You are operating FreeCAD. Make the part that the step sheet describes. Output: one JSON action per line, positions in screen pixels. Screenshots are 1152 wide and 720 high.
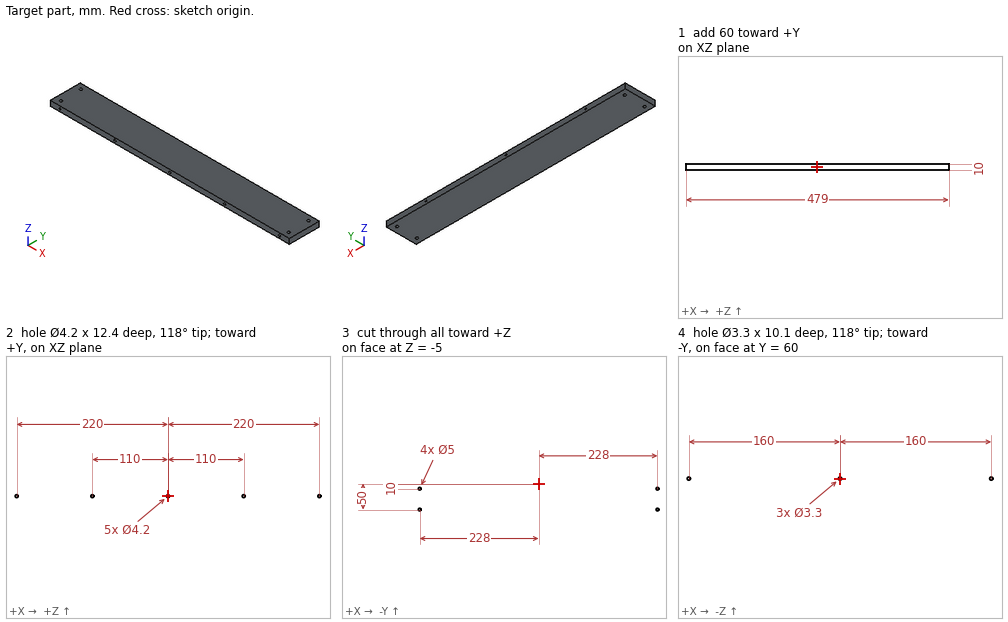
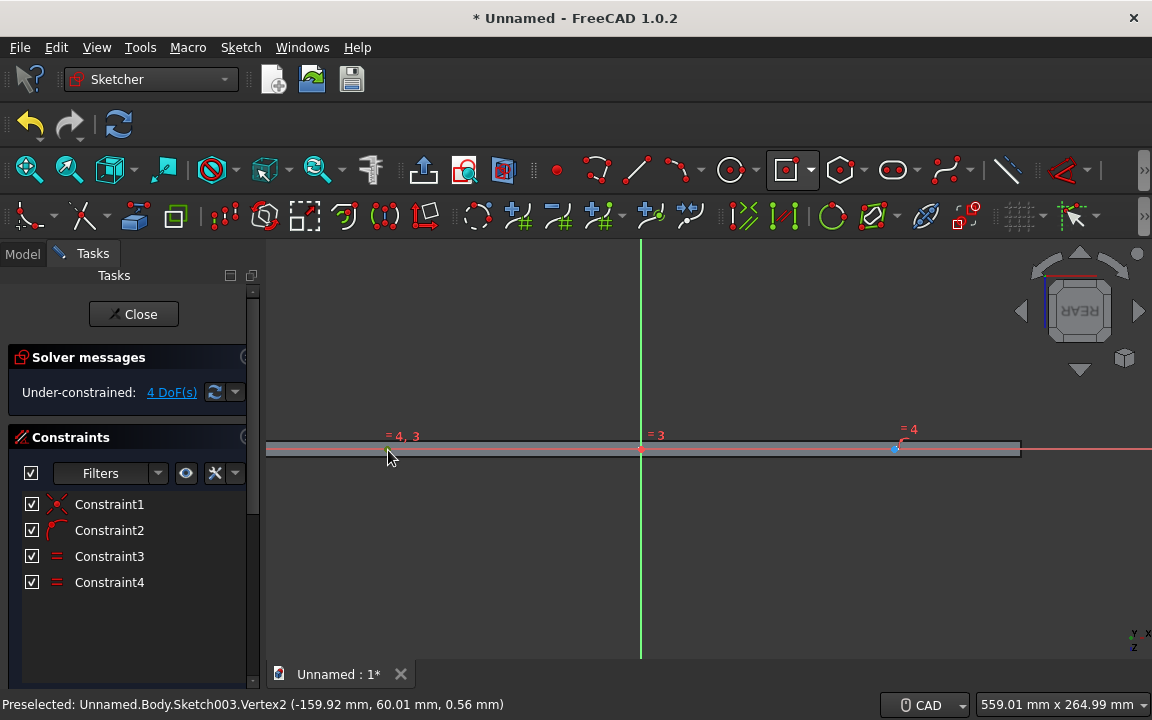
{"action": "left_click", "coordinate": [344, 449]}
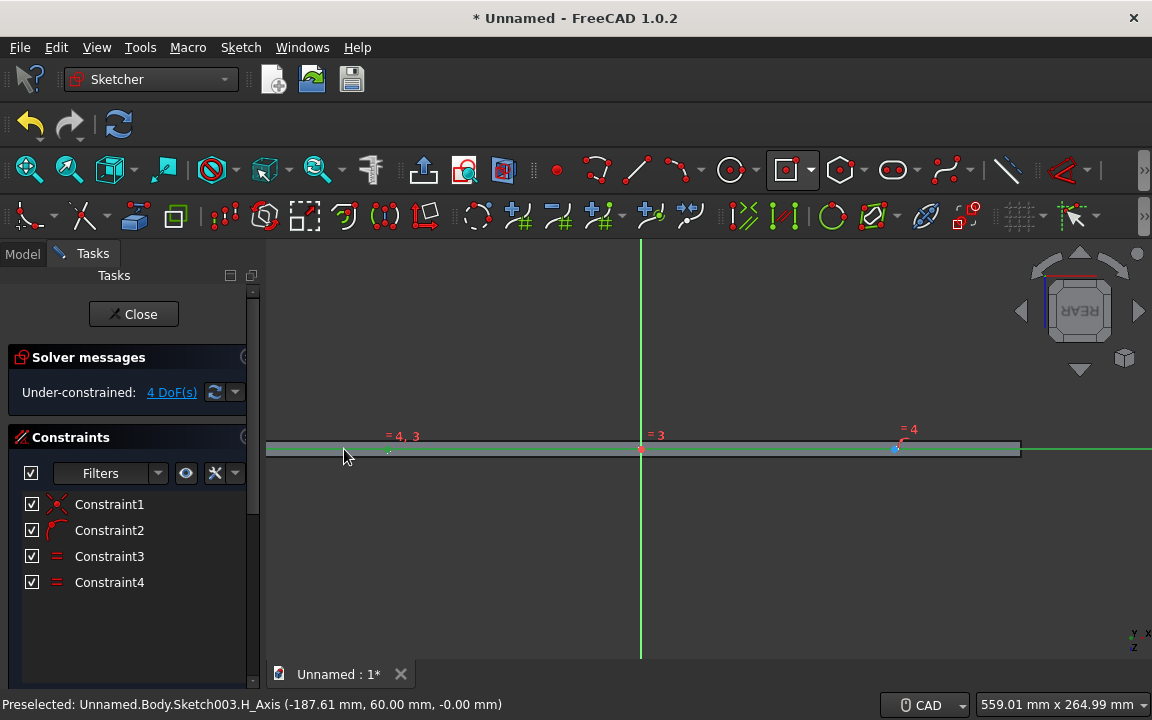
{"action": "key", "text": "c"}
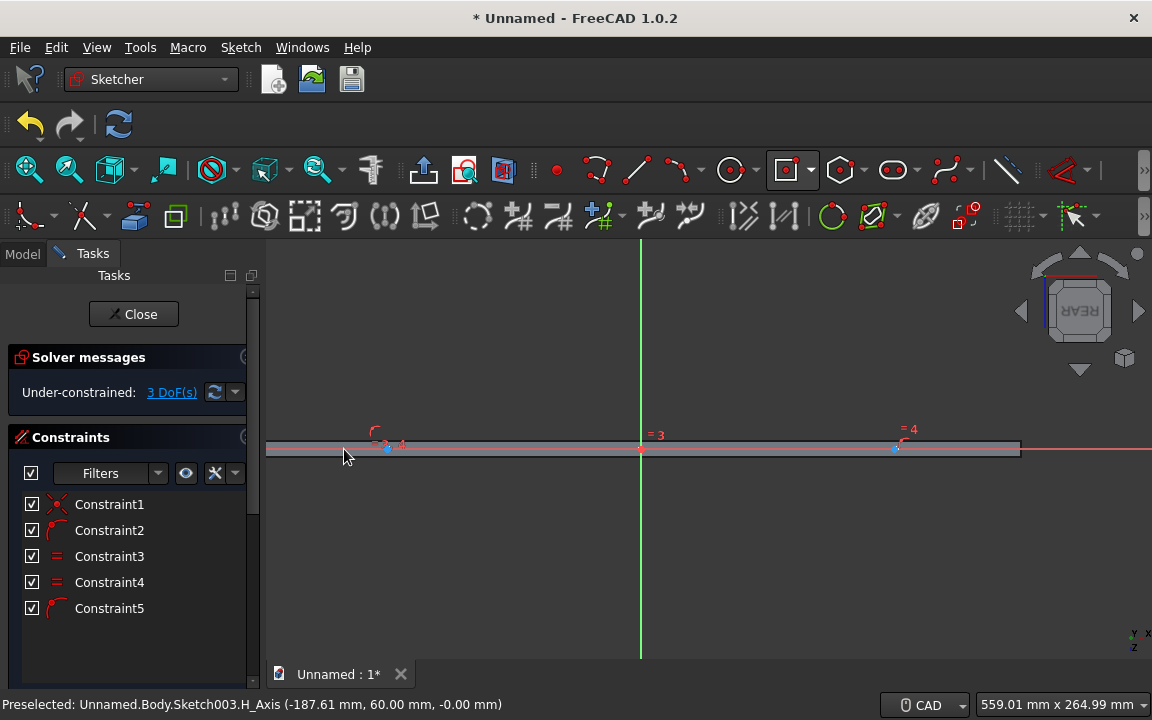
{"action": "key", "text": "d"}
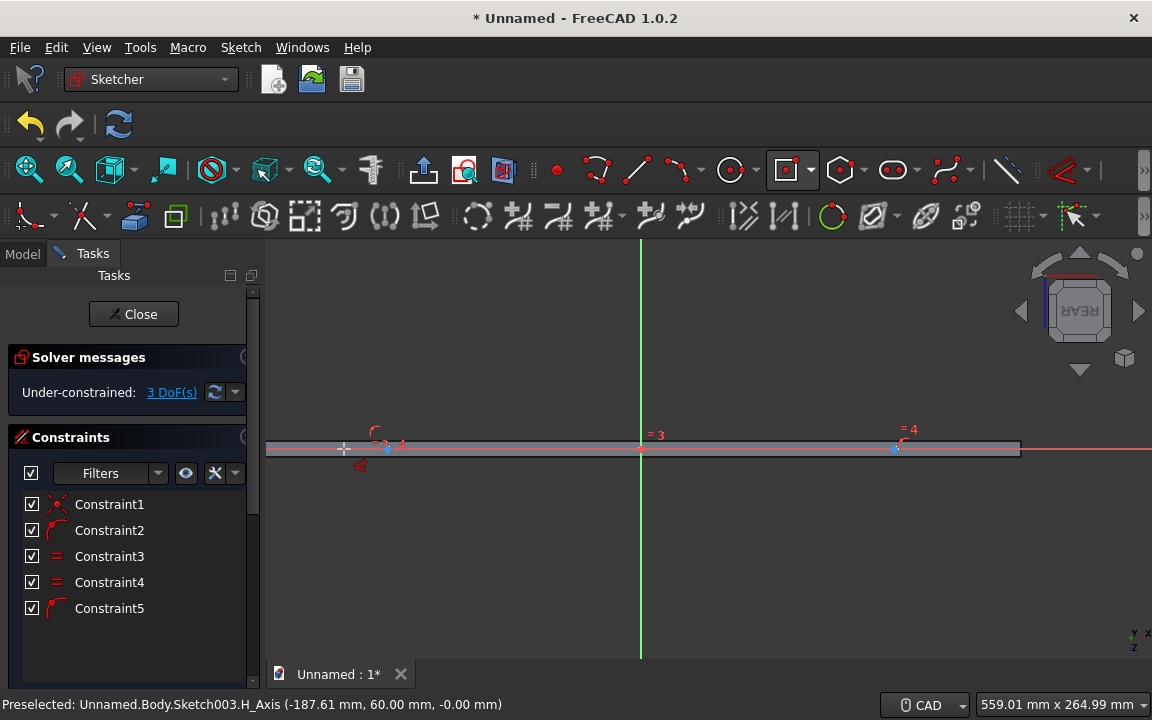
{"action": "scroll", "coordinate": [640, 447], "scroll_direction": "up", "scroll_amount": 11}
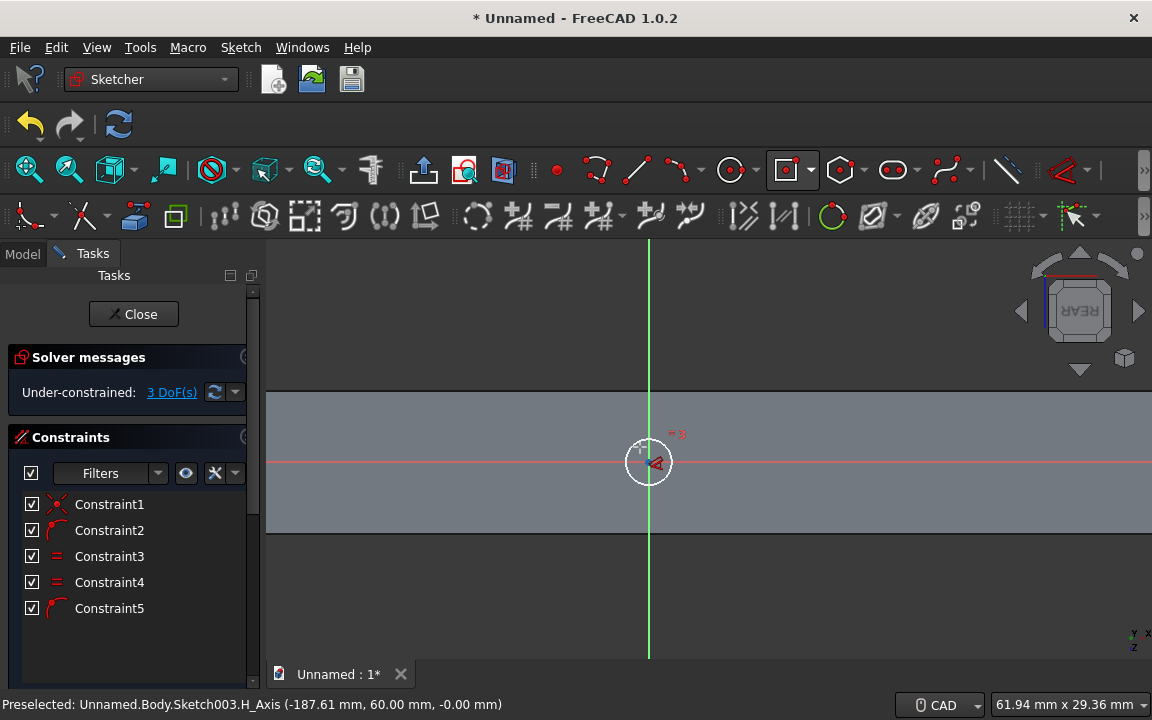
{"action": "left_click", "coordinate": [633, 446]}
{"action": "left_click", "coordinate": [611, 423]}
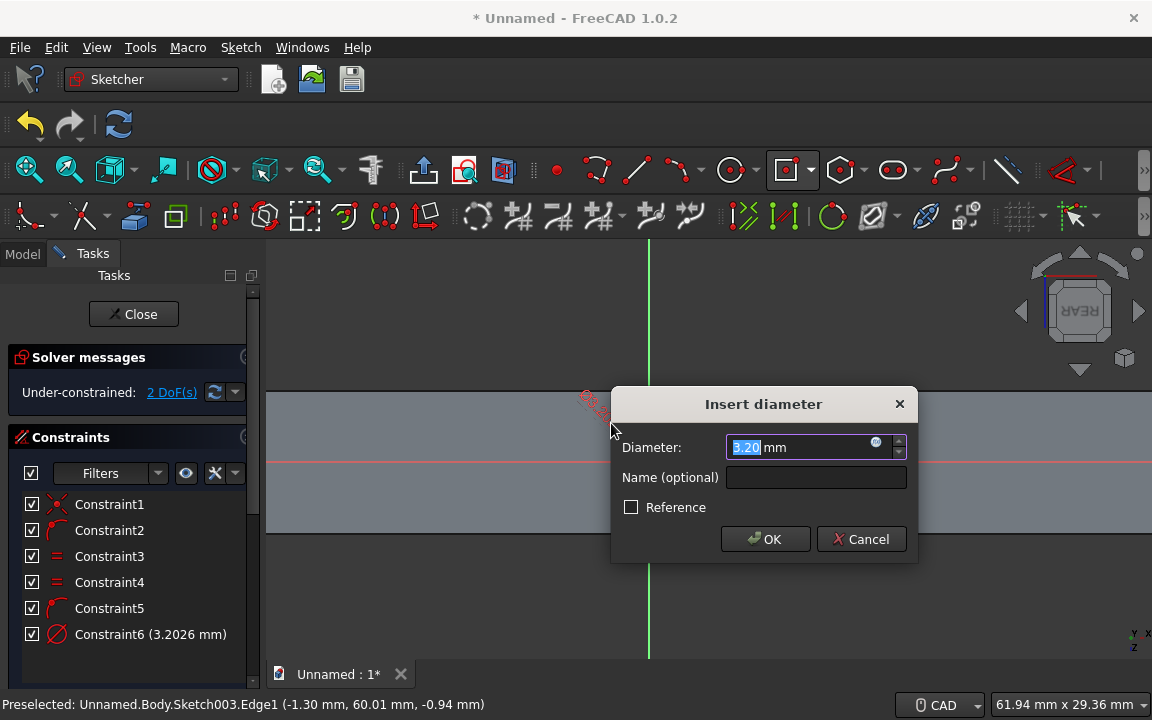
{"action": "type", "text": "3.3"}
{"action": "key", "text": "Return"}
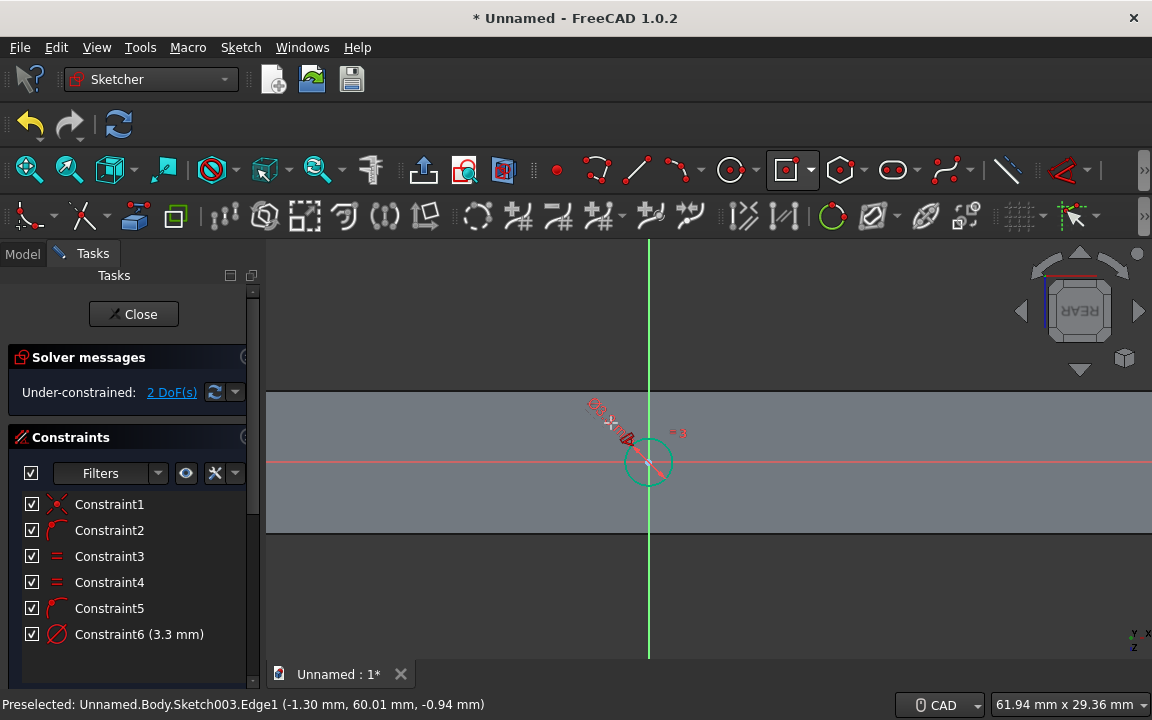
{"action": "scroll", "coordinate": [639, 447], "scroll_direction": "down", "scroll_amount": 11}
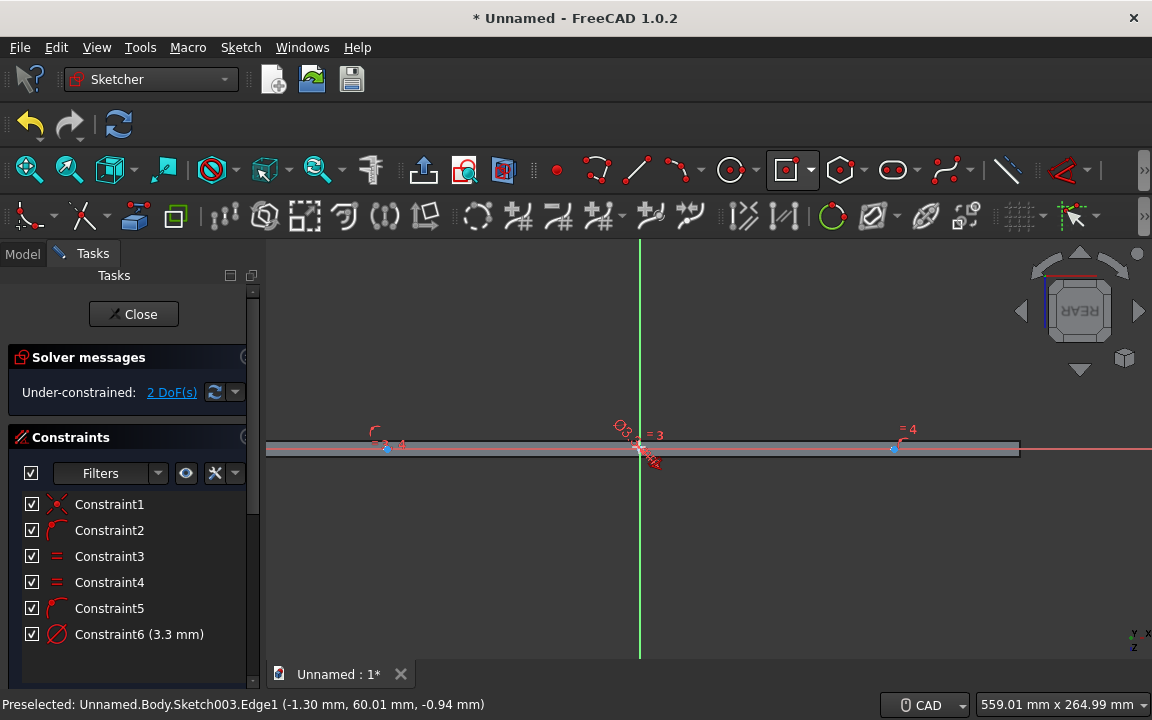
{"action": "left_click", "coordinate": [387, 449]}
{"action": "left_click", "coordinate": [514, 483]}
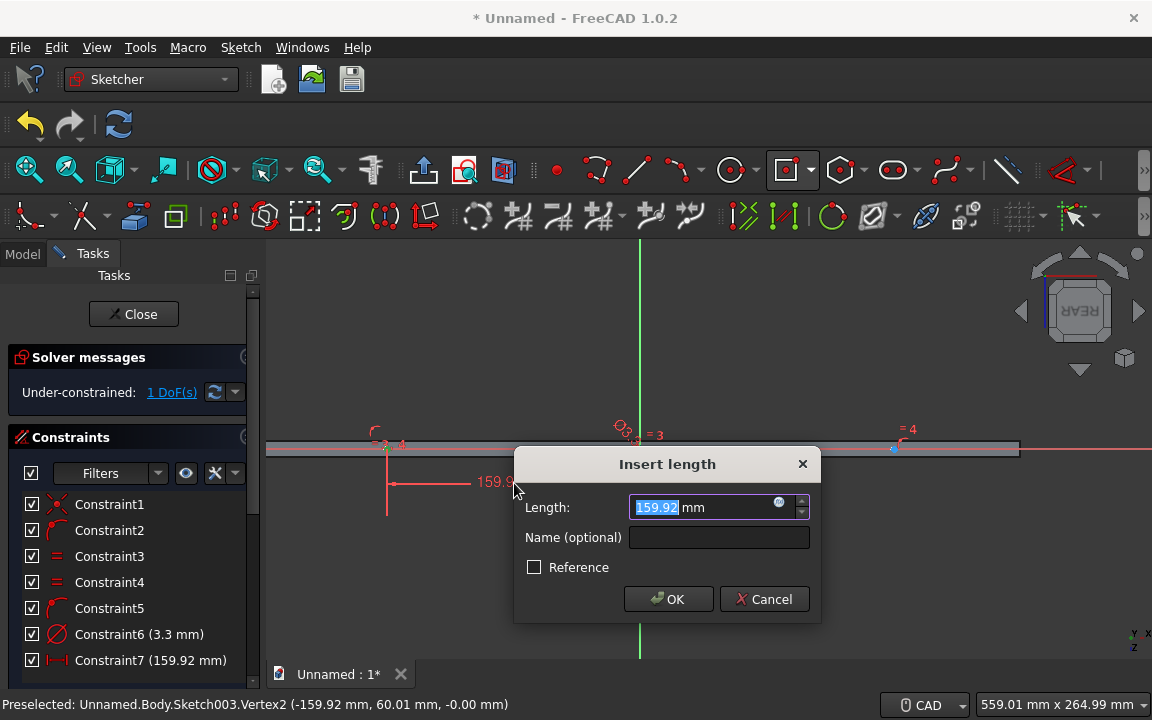
{"action": "type", "text": "160"}
{"action": "key", "text": "Return"}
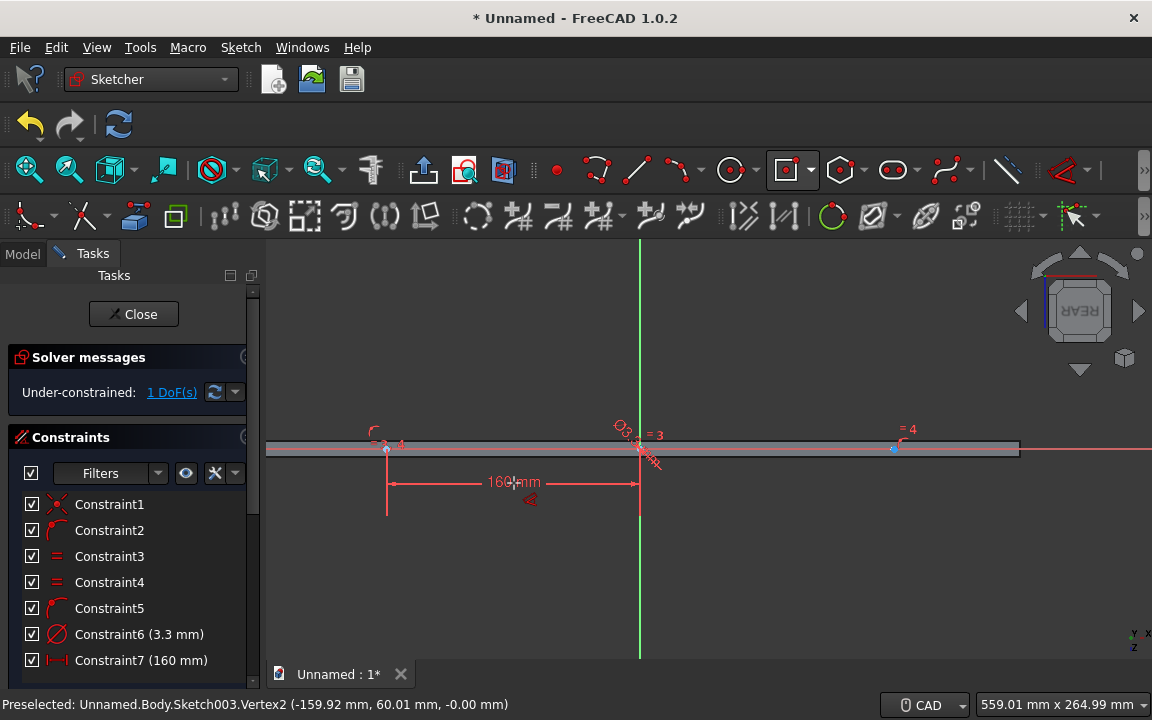
{"action": "left_click", "coordinate": [894, 449]}
{"action": "left_click", "coordinate": [767, 483]}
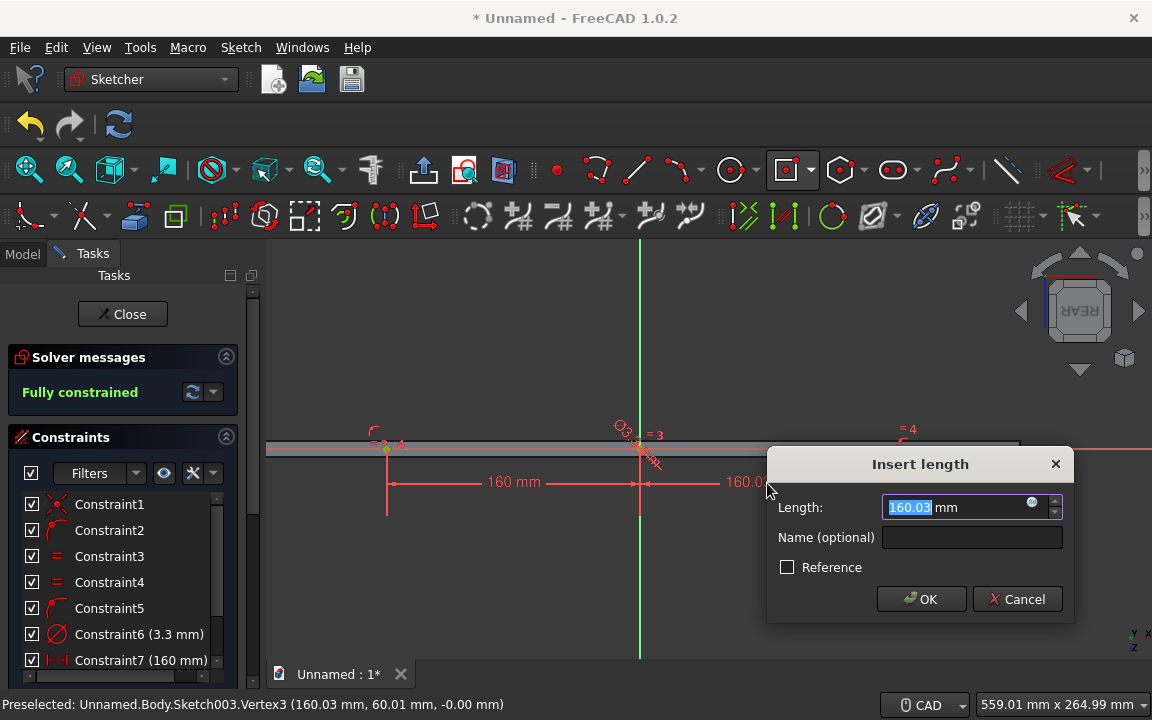
{"action": "type", "text": "160"}
{"action": "key", "text": "Return"}
{"action": "key", "text": "Escape"}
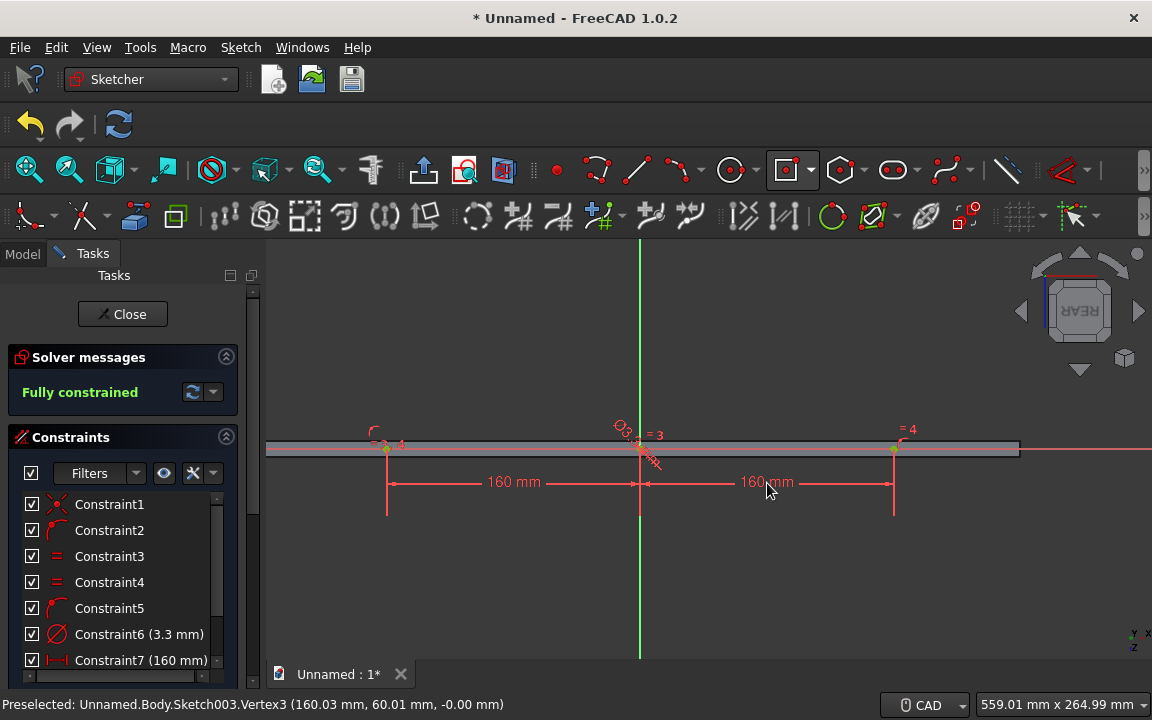
{"action": "left_click", "coordinate": [123, 314]}